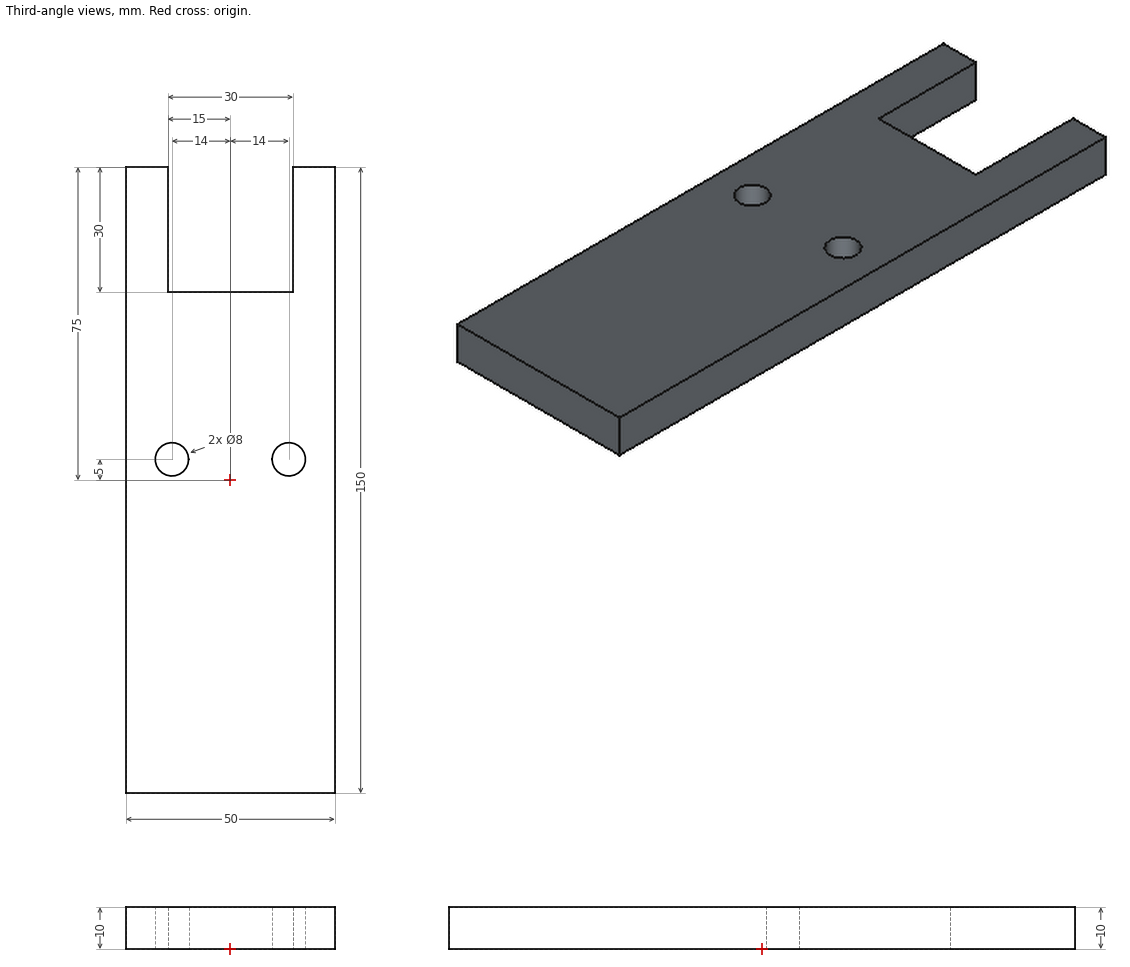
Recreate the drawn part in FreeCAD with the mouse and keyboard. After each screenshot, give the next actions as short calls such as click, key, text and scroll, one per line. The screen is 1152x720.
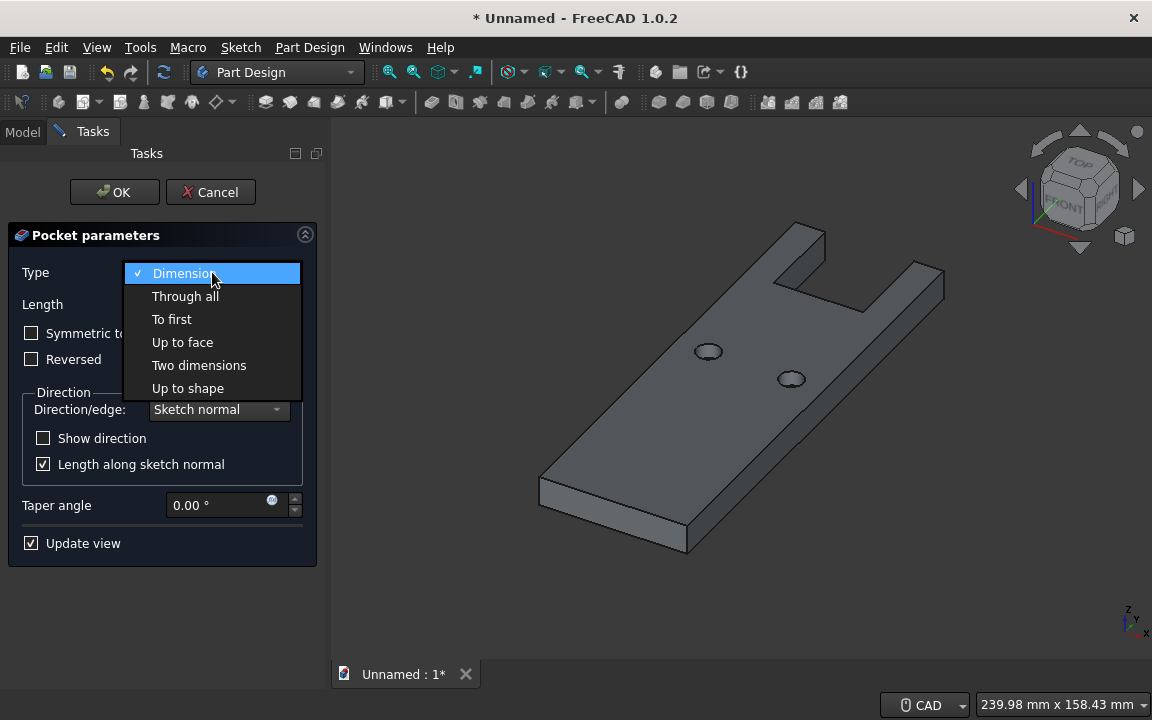
click(212, 296)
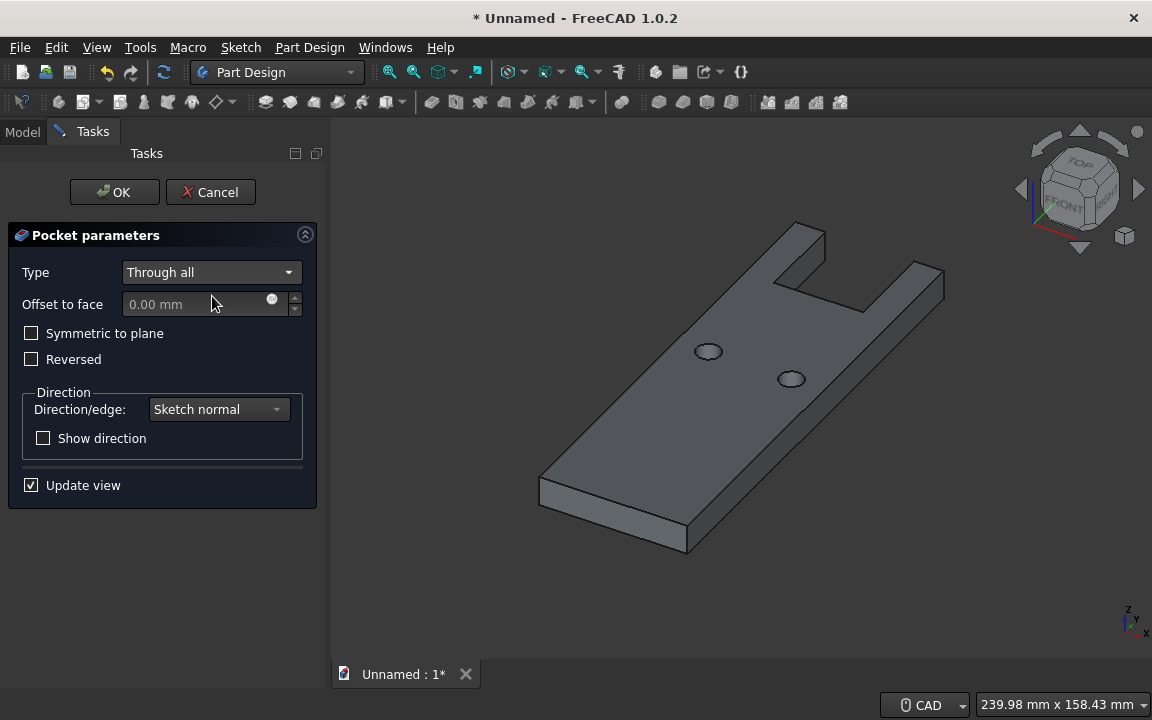
click(115, 192)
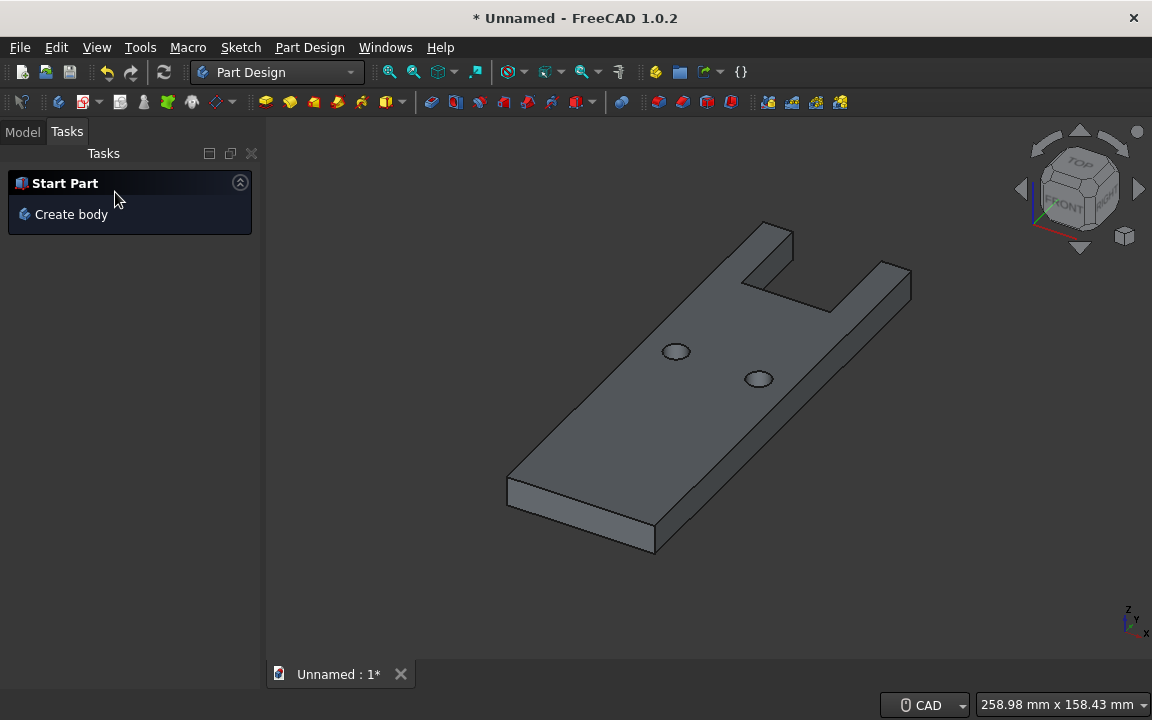
key(0)